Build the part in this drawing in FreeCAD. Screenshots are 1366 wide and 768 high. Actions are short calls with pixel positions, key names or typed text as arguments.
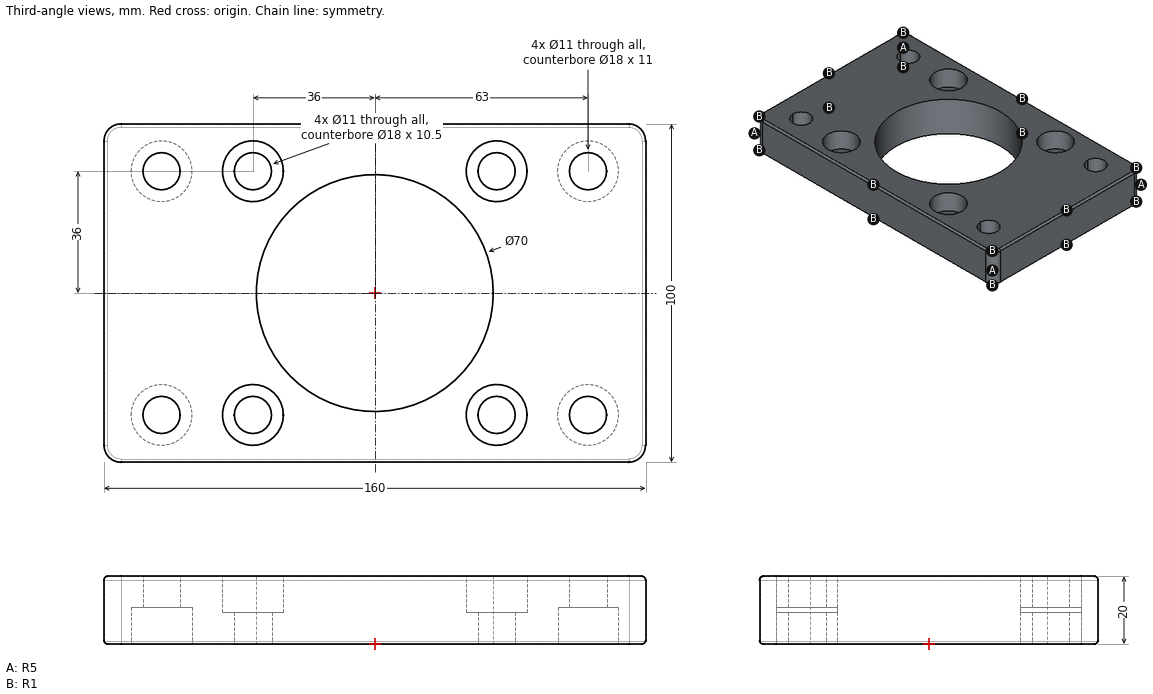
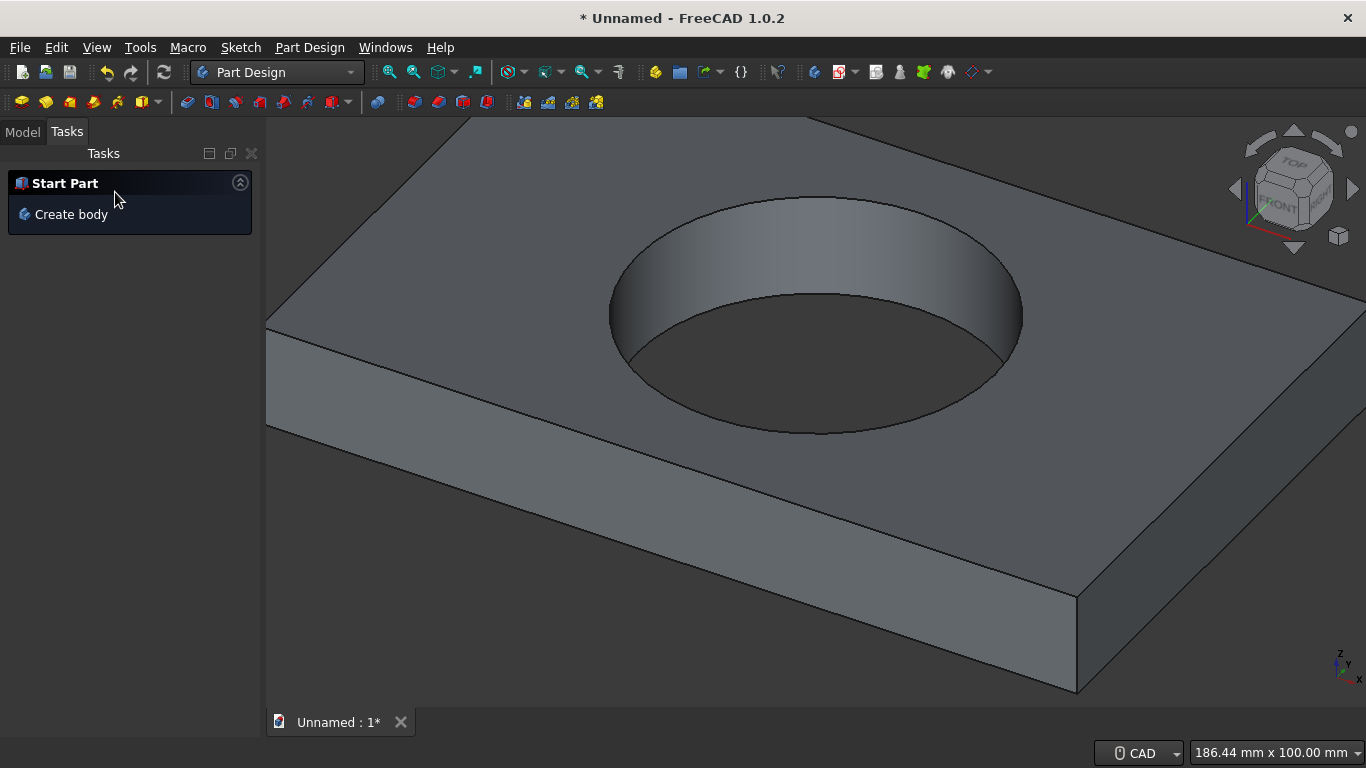
key(v)
key(f)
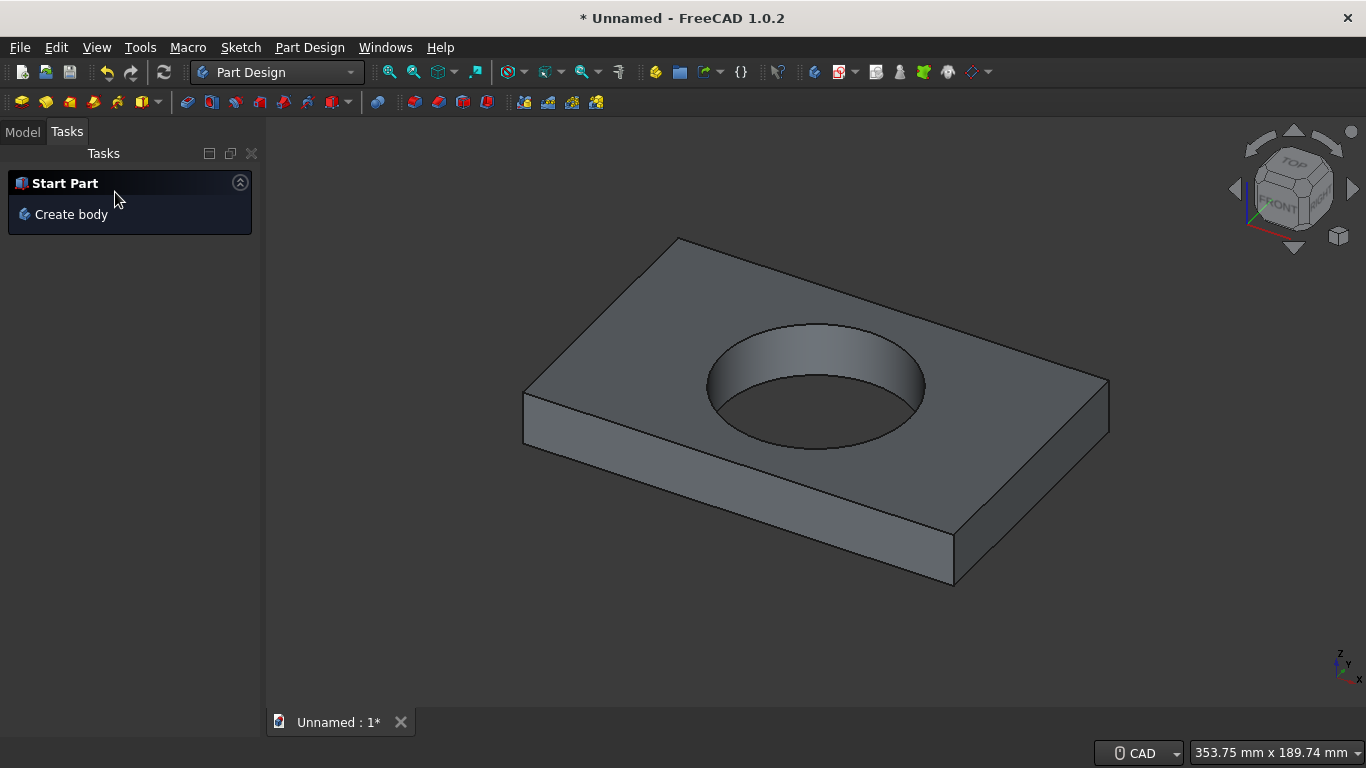
click(954, 560)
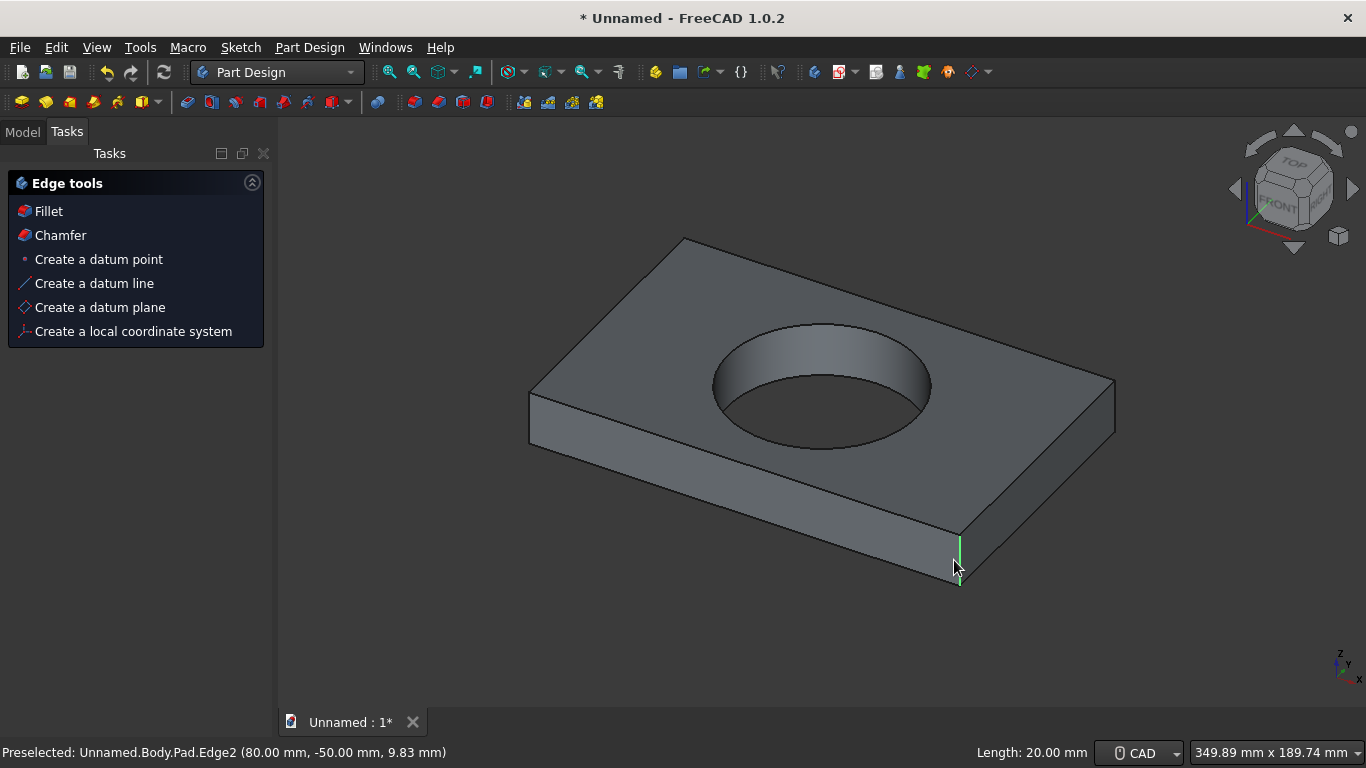
key(0)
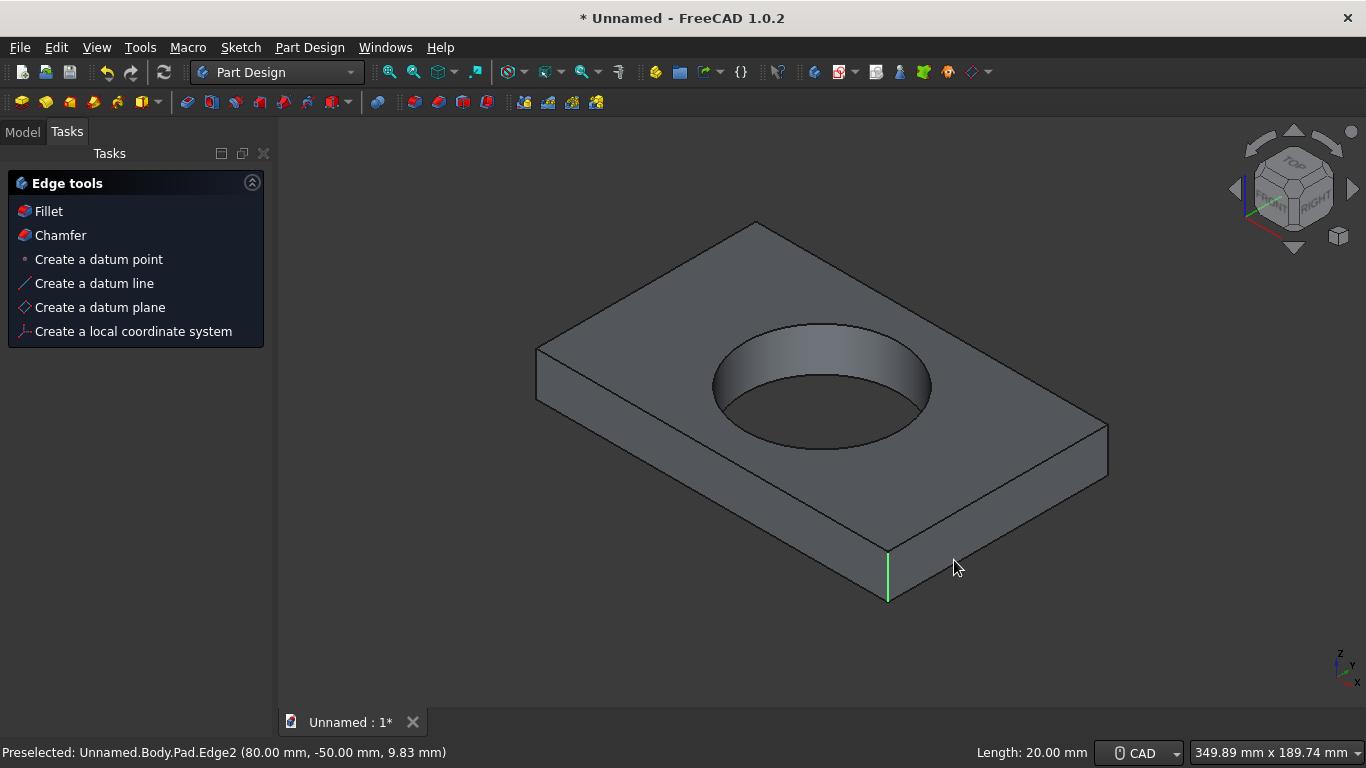
key(2)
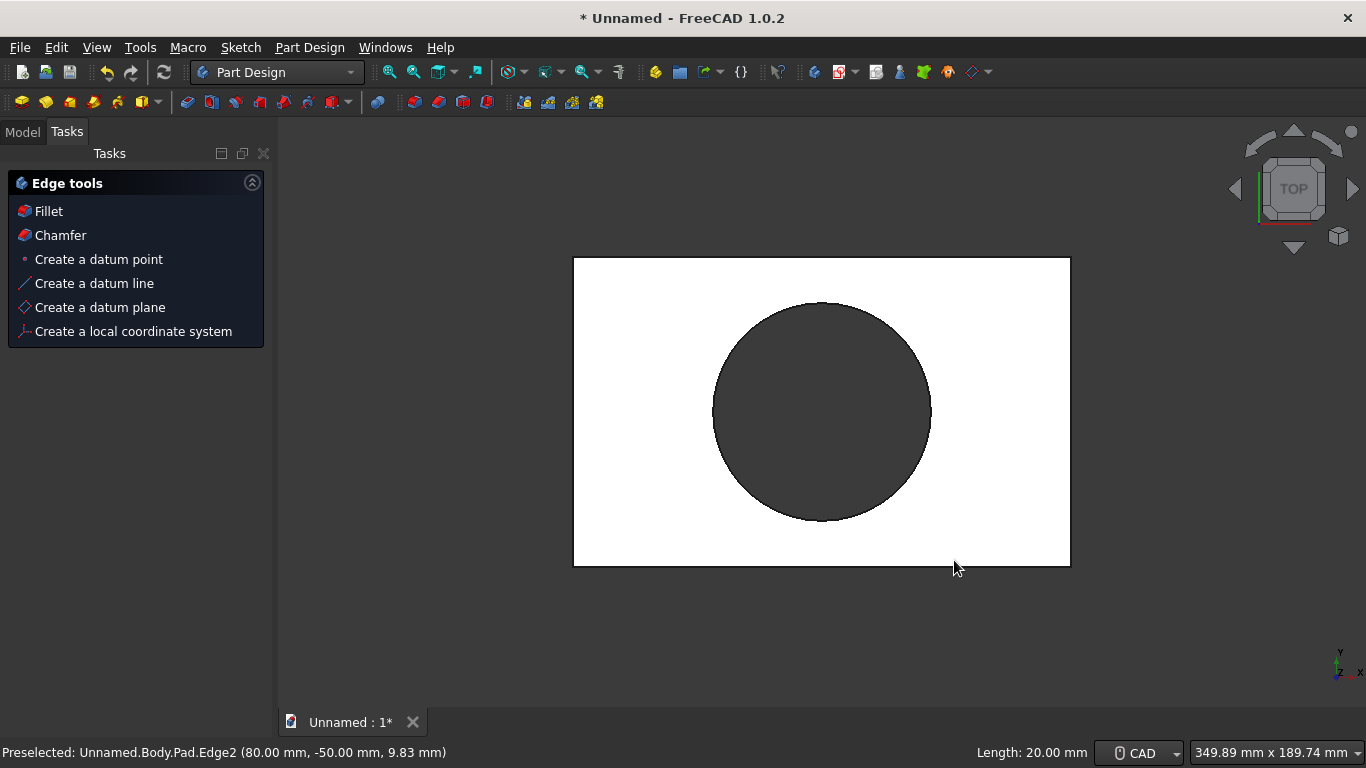
key(1)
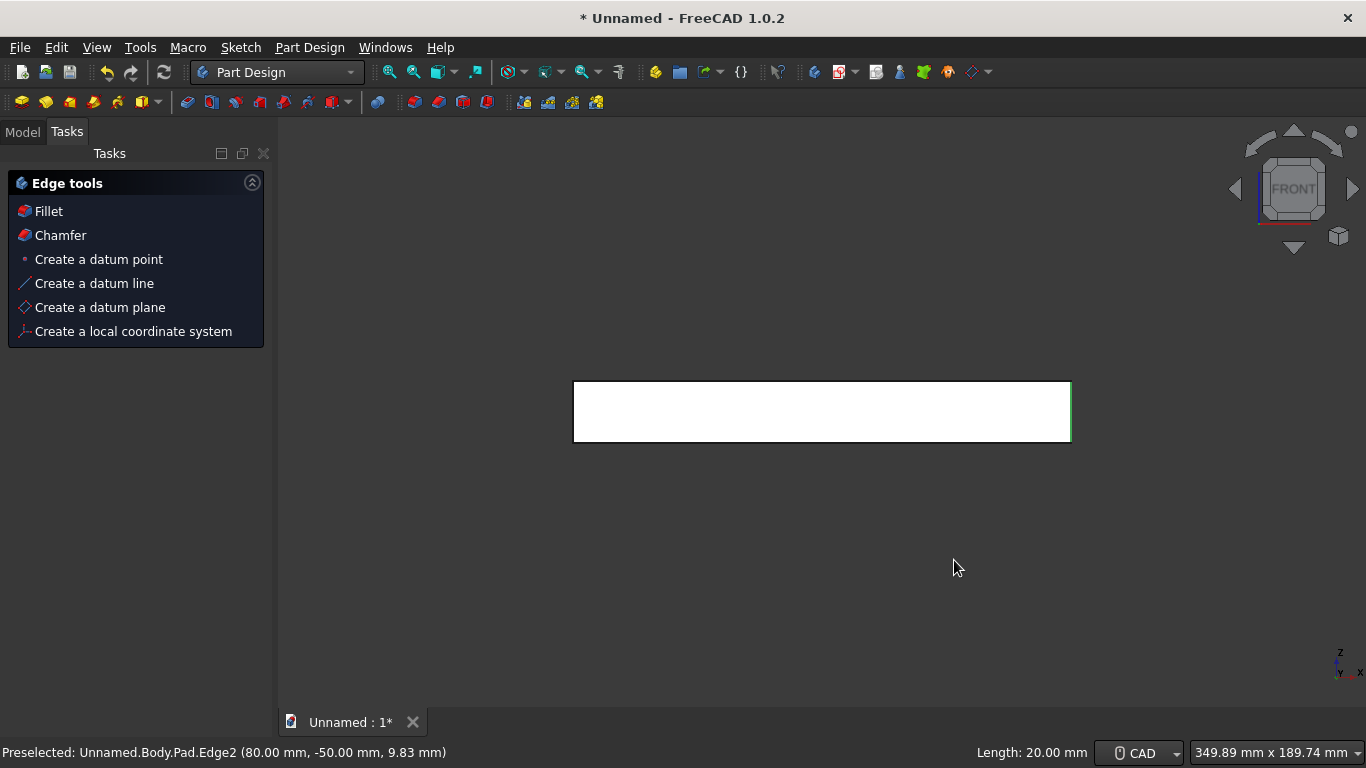
click(573, 411, ctrl)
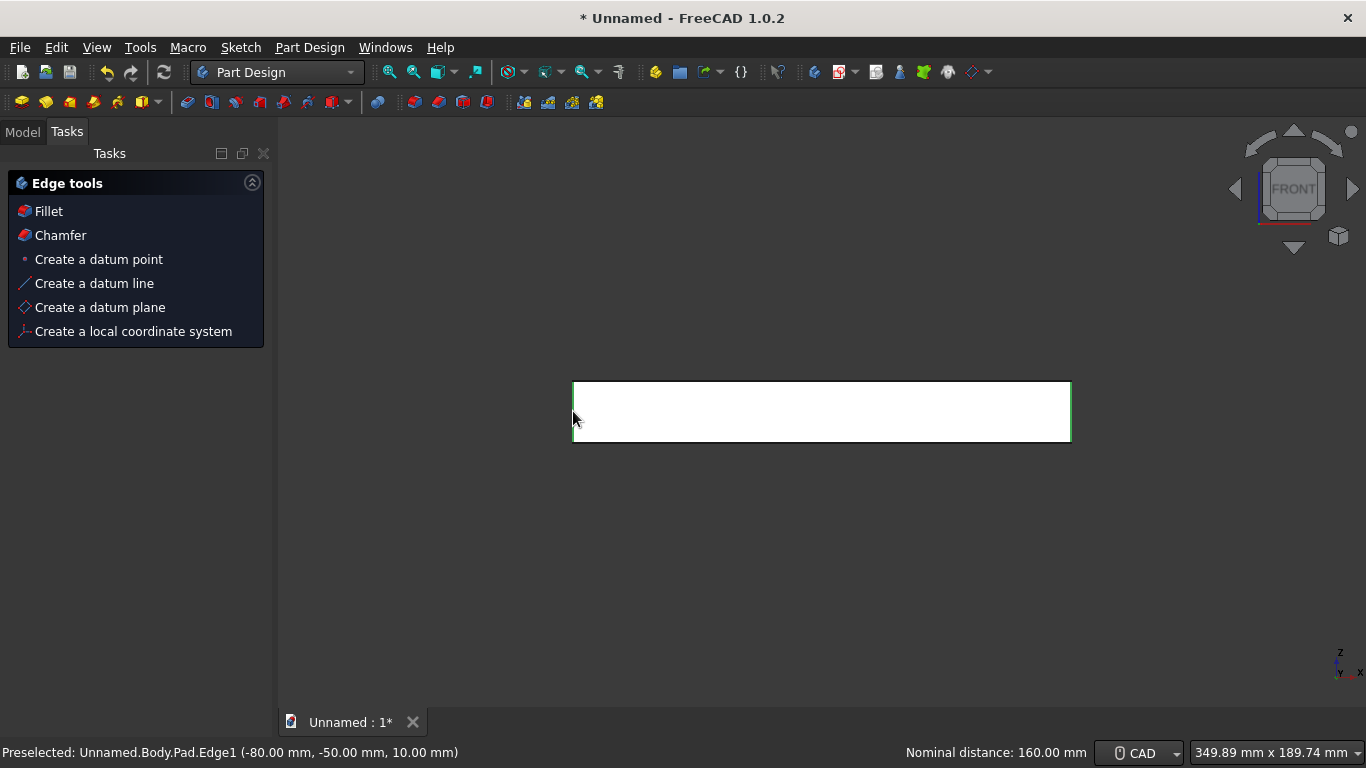
key(3)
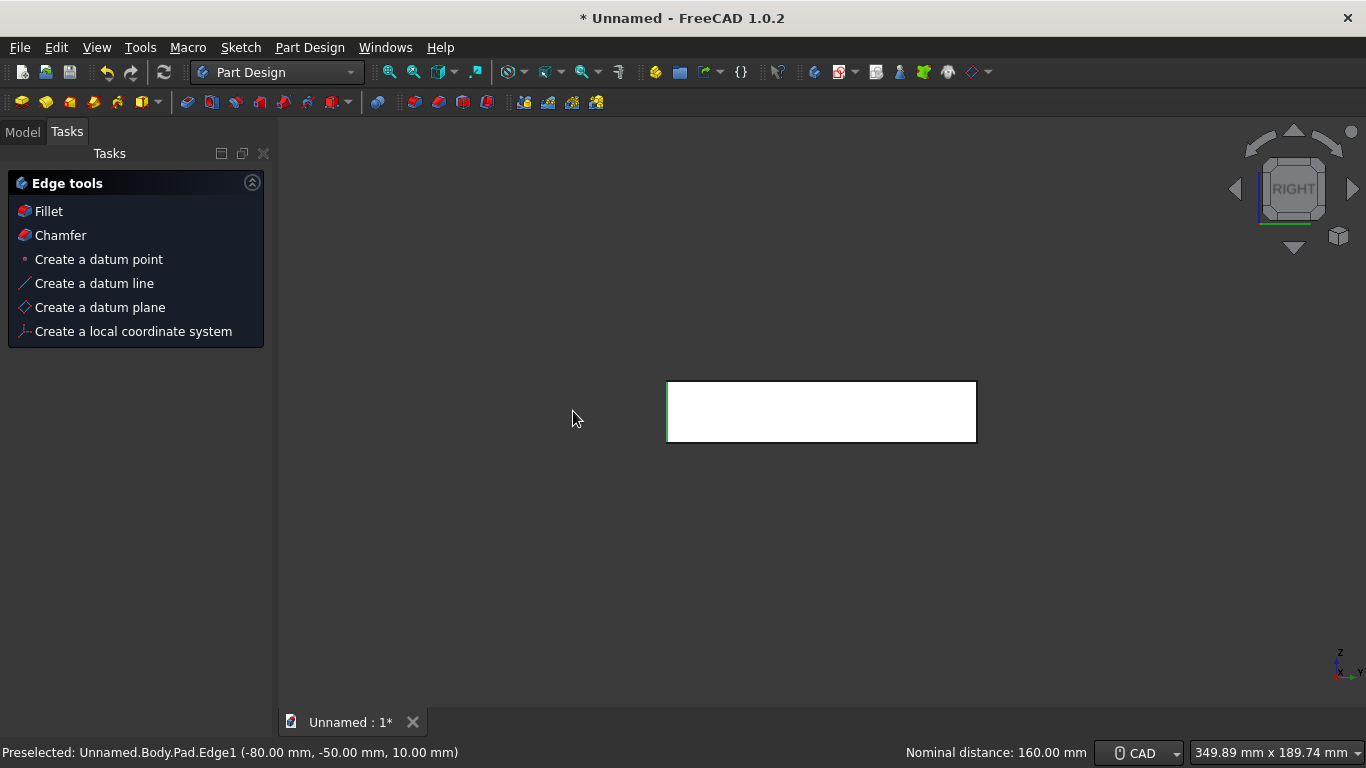
key(v)
key(f)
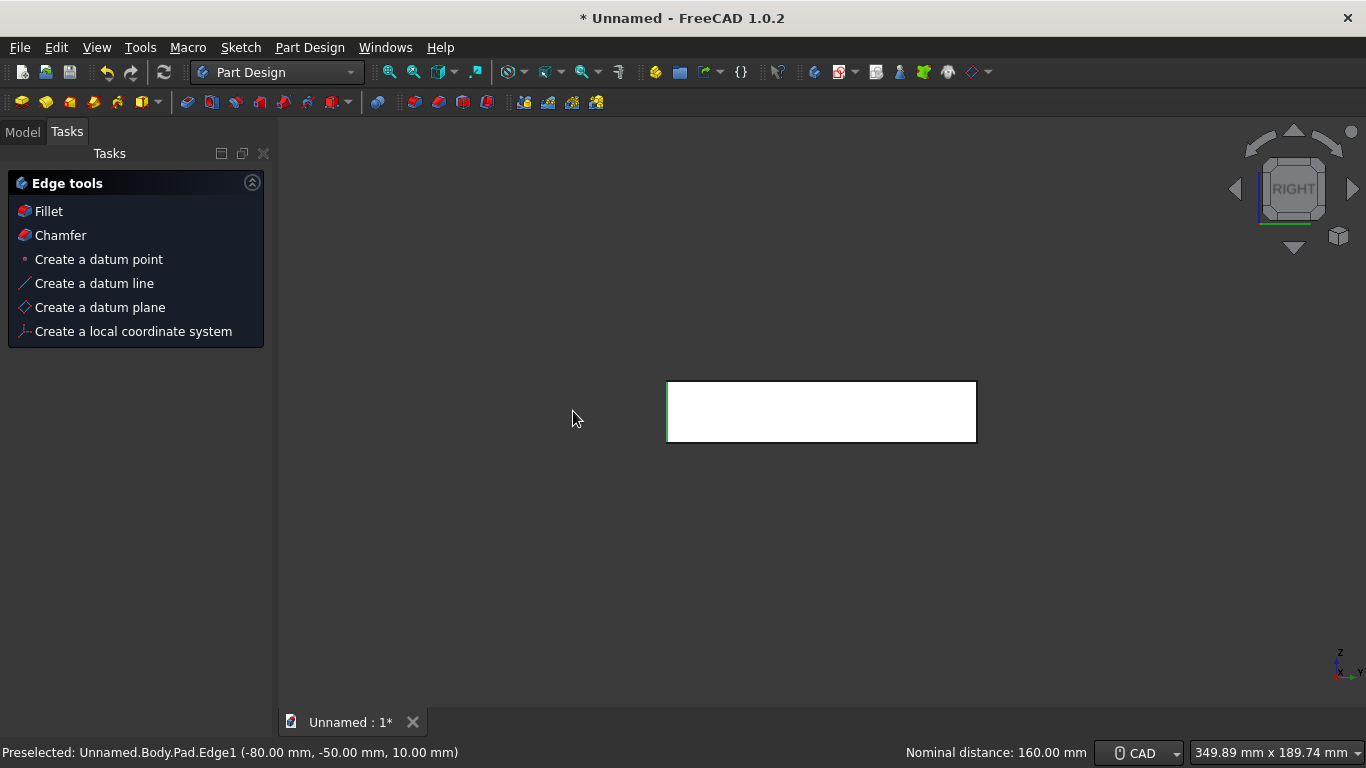
click(977, 411, ctrl)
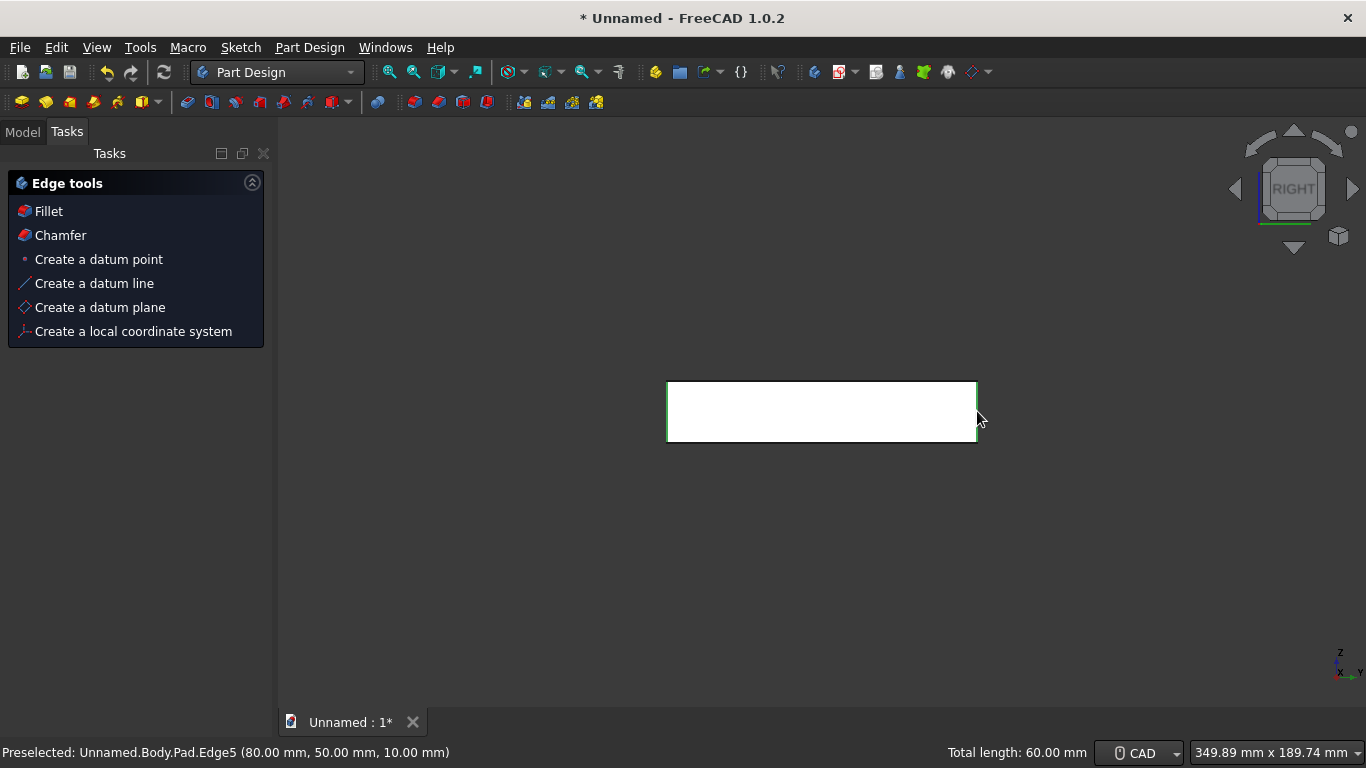
key(5)